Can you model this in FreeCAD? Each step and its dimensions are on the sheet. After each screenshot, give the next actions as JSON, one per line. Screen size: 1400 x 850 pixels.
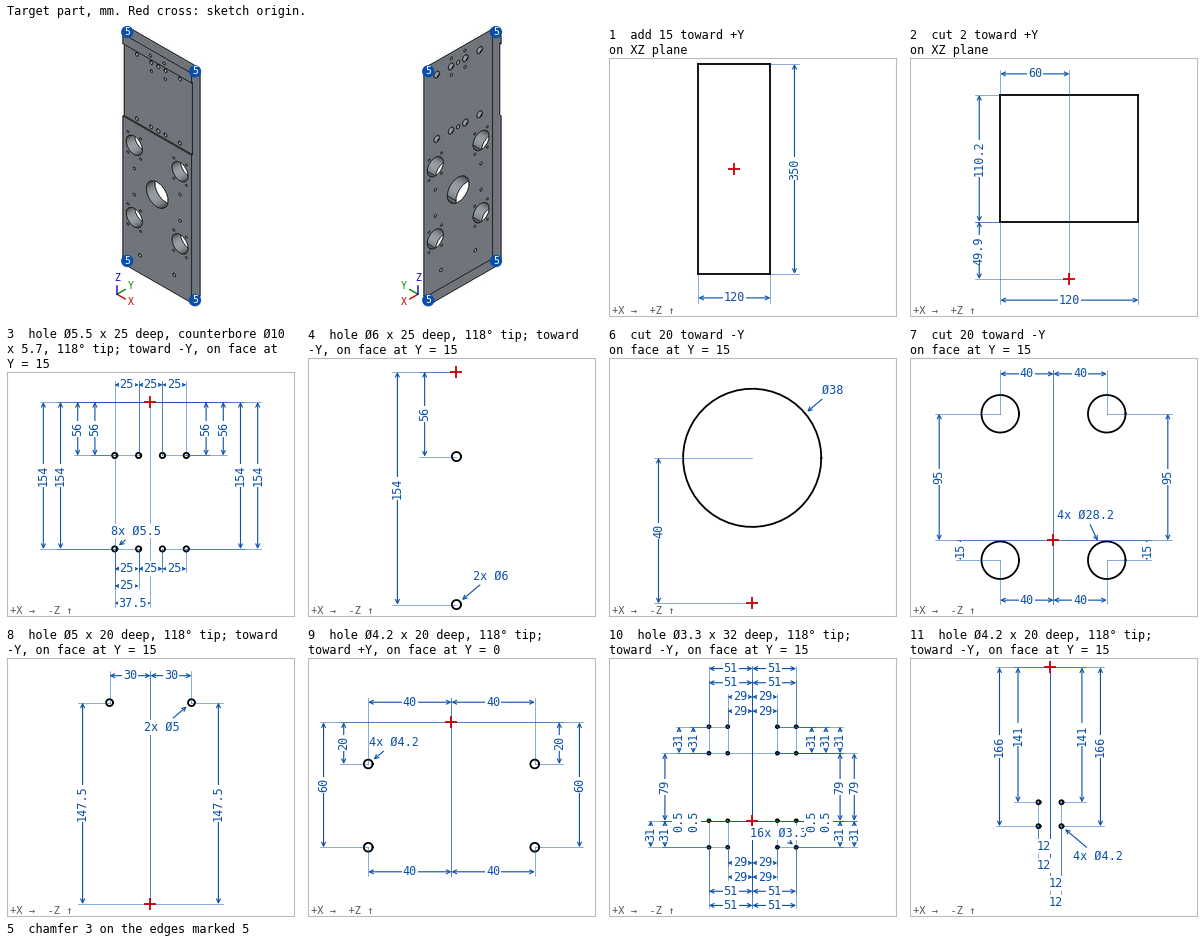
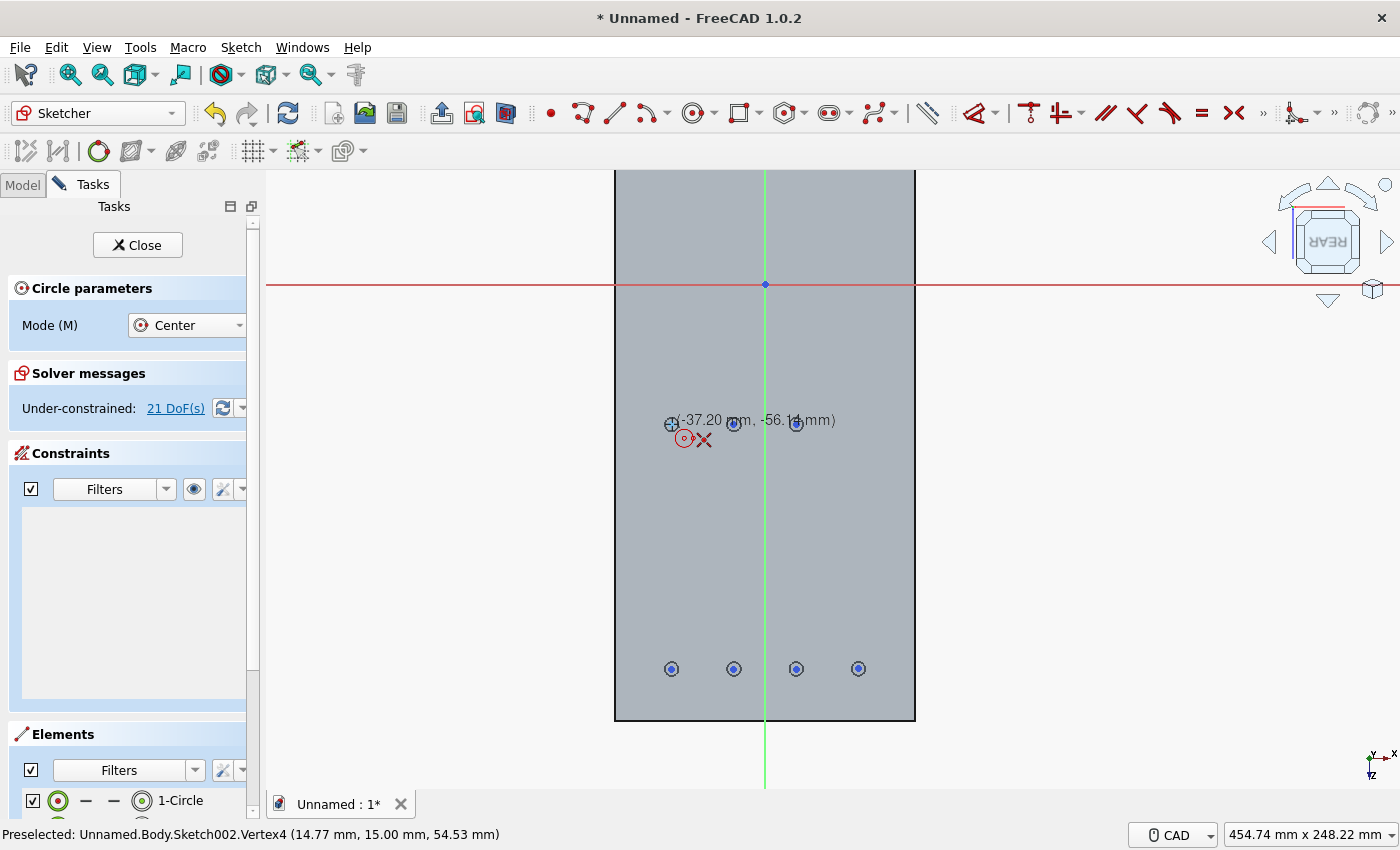
{"action": "scroll", "coordinate": [859, 424], "scroll_direction": "up", "scroll_amount": 6}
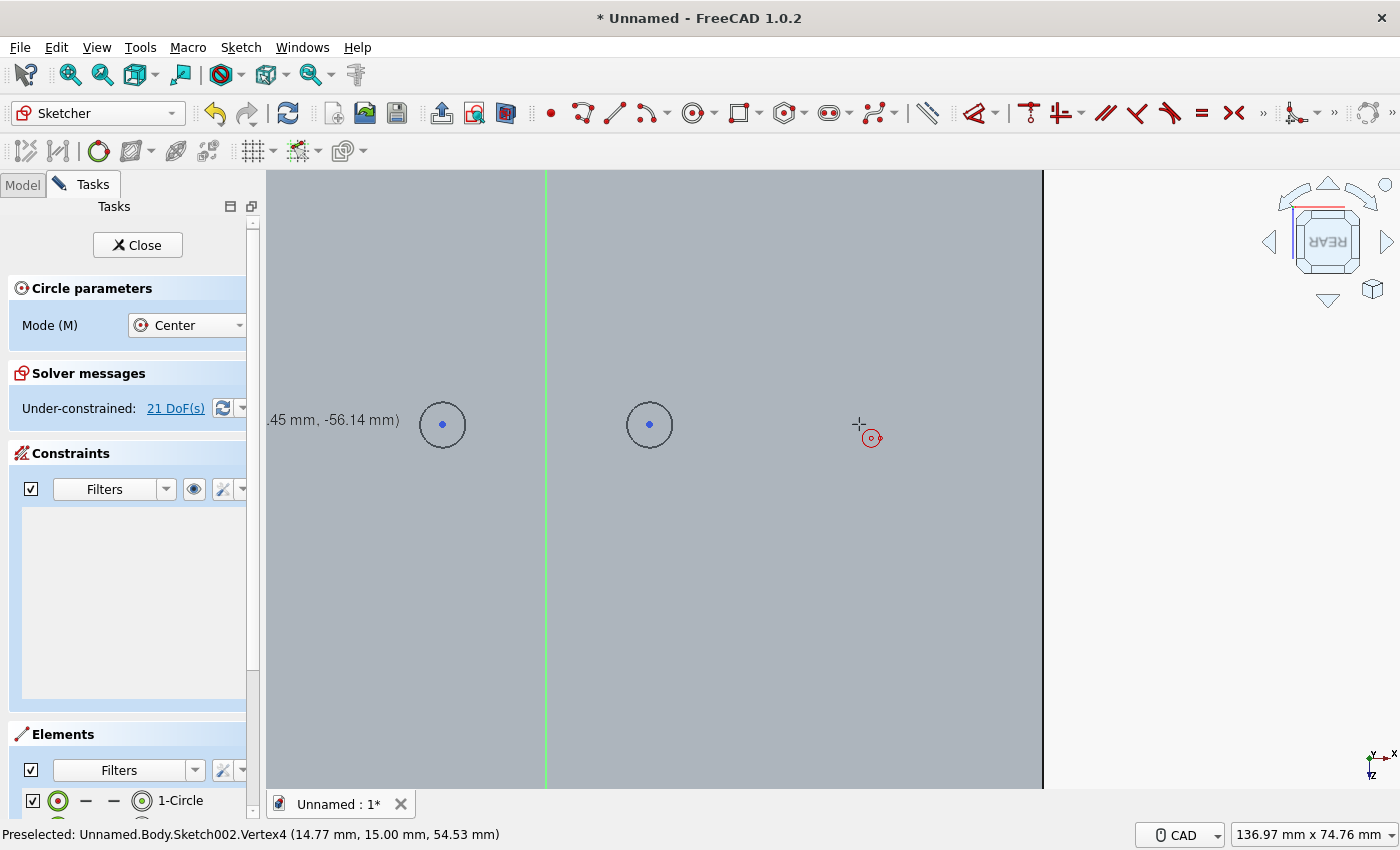
{"action": "left_click", "coordinate": [856, 424]}
{"action": "left_click", "coordinate": [872, 408]}
{"action": "key", "text": "Escape"}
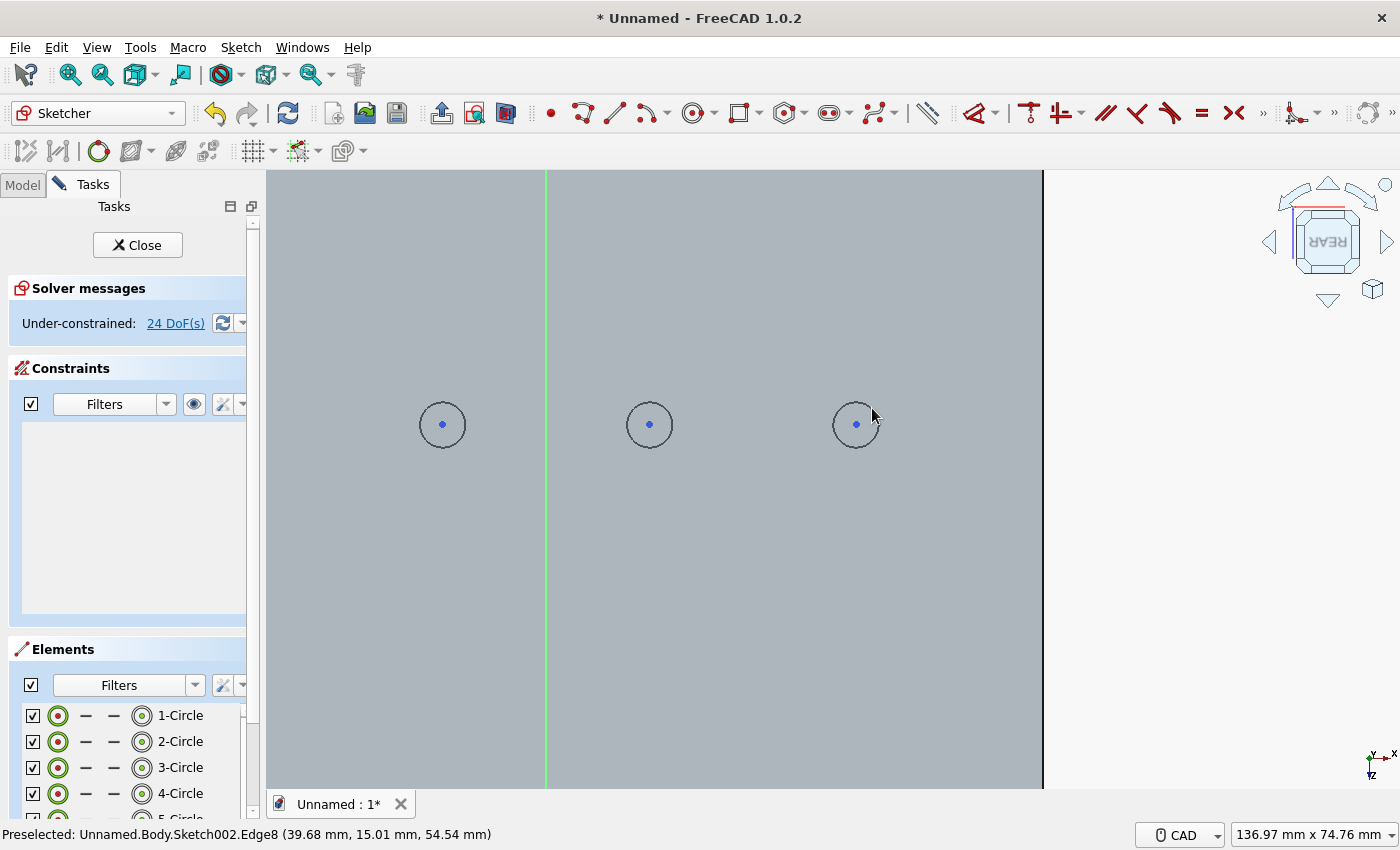
{"action": "scroll", "coordinate": [859, 424], "scroll_direction": "down", "scroll_amount": 6}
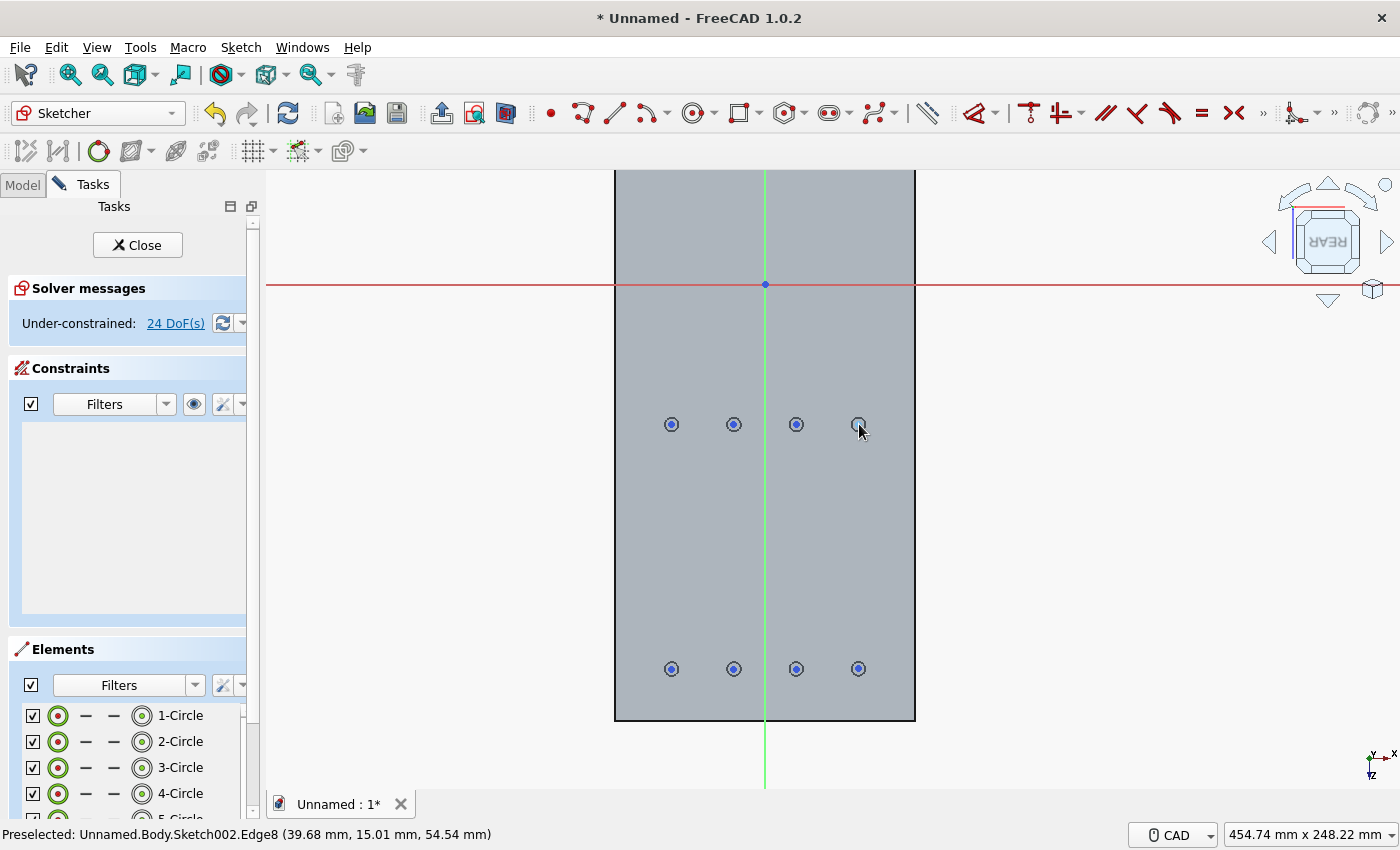
{"action": "scroll", "coordinate": [676, 664], "scroll_direction": "up", "scroll_amount": 4}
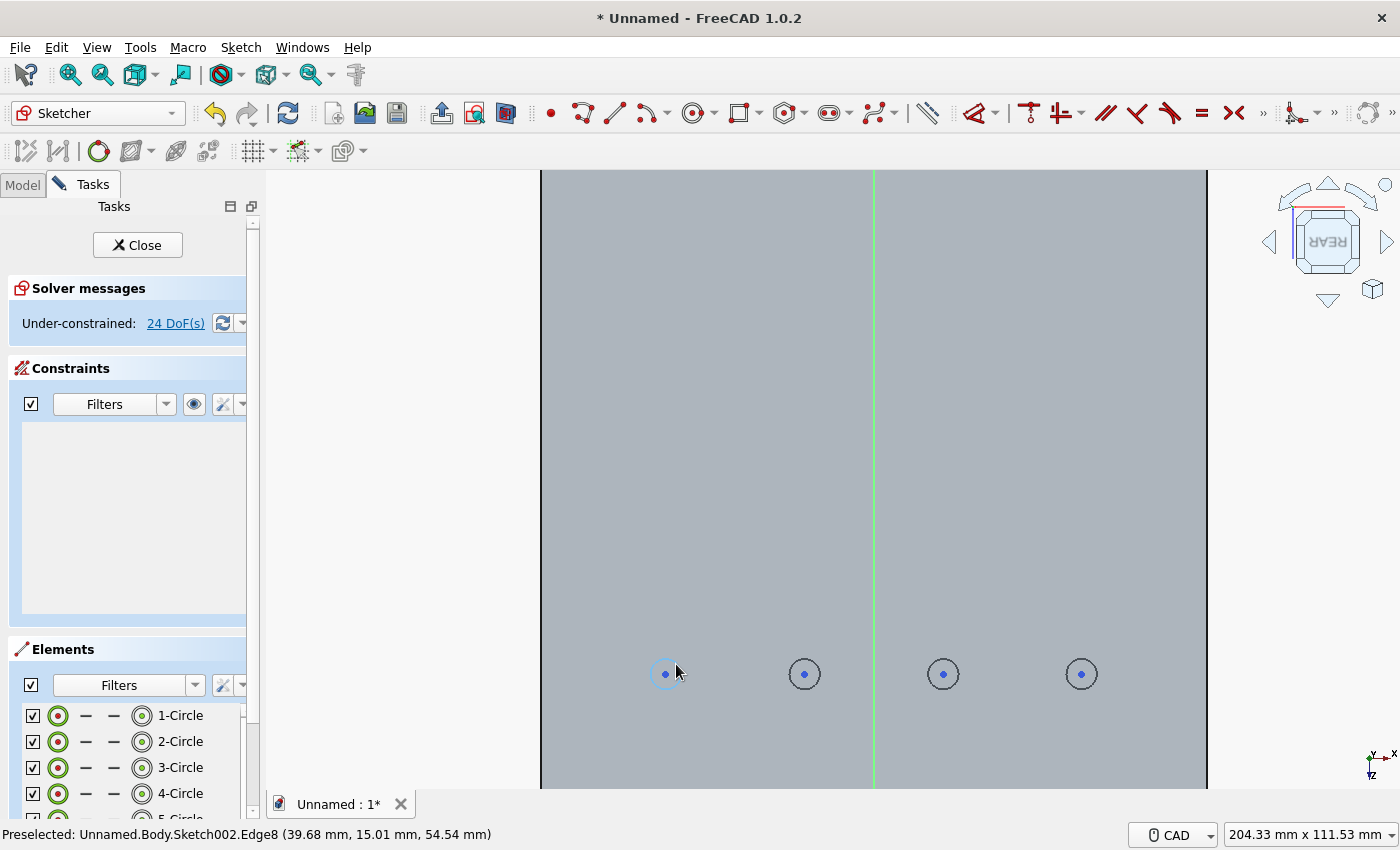
{"action": "left_click", "coordinate": [677, 663]}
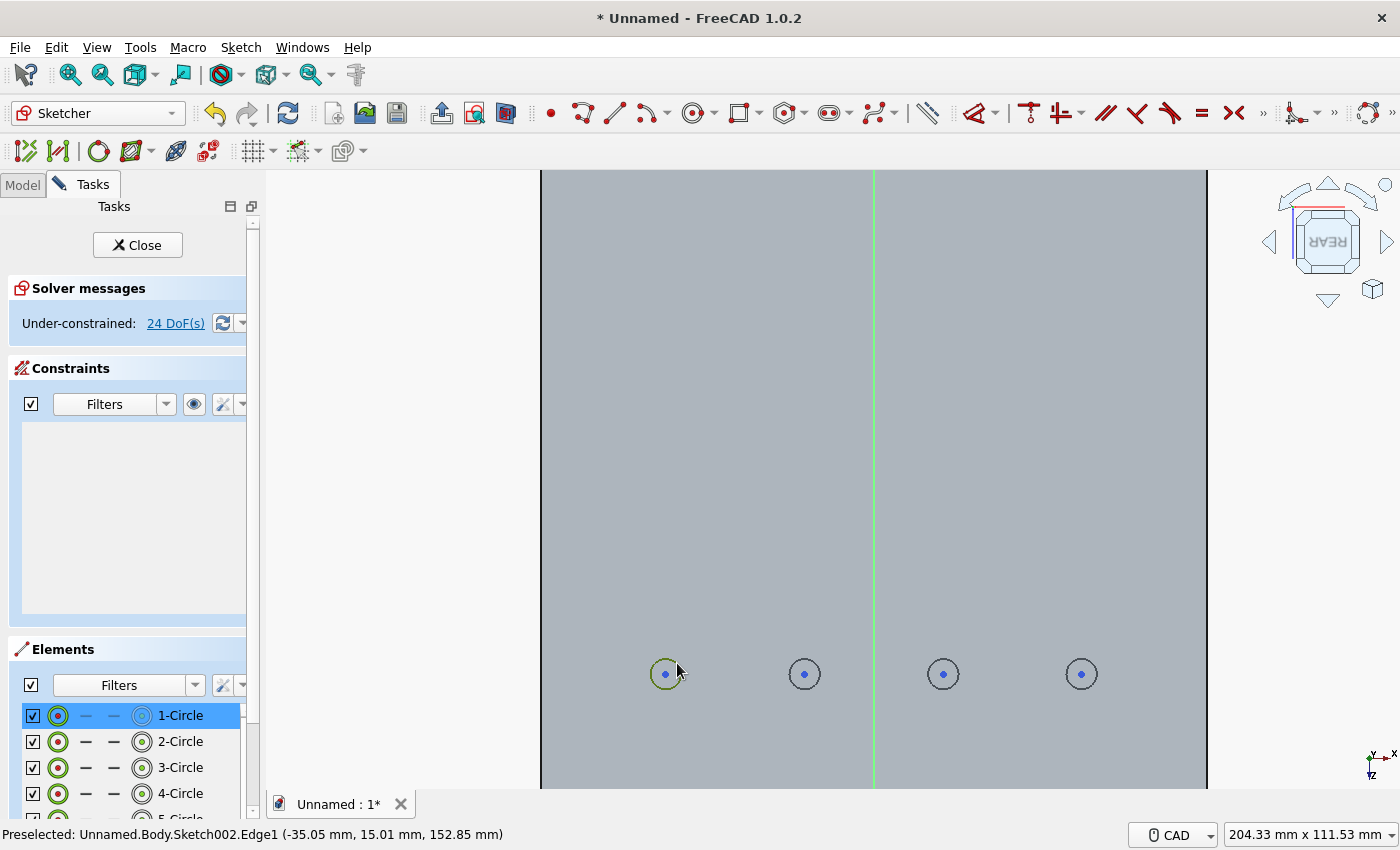
{"action": "left_click", "coordinate": [815, 663]}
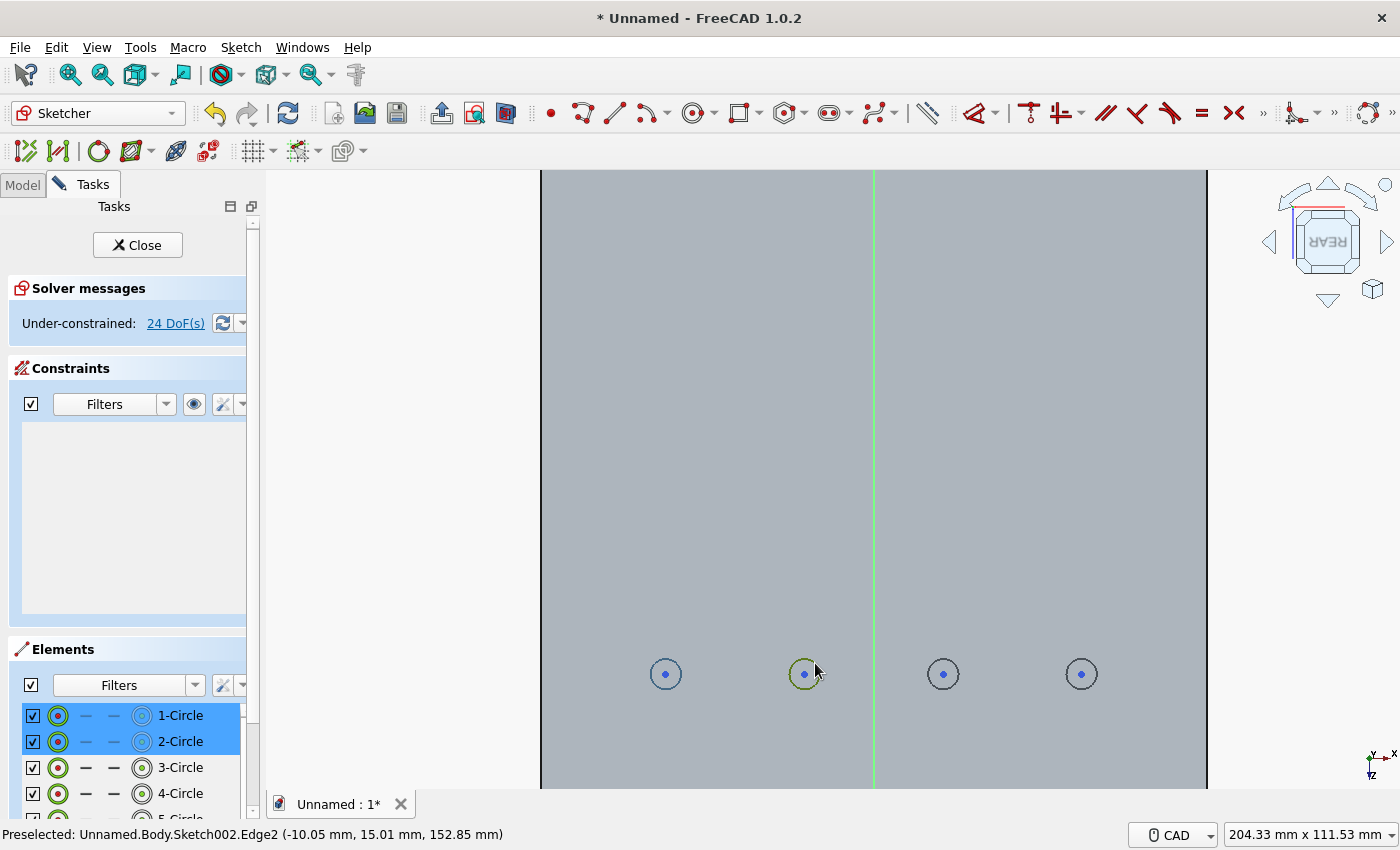
{"action": "left_click", "coordinate": [954, 663]}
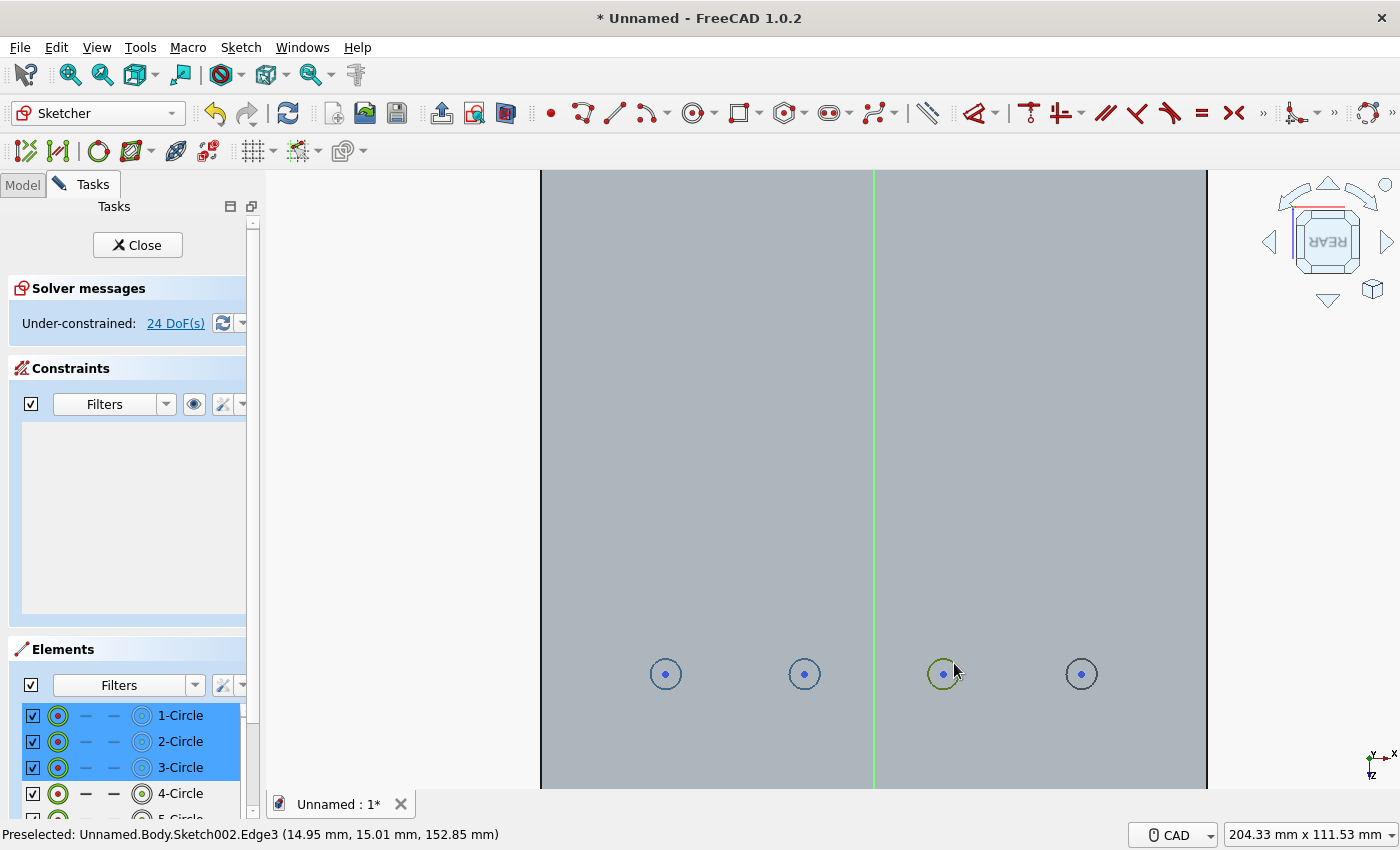
{"action": "left_click", "coordinate": [1092, 663]}